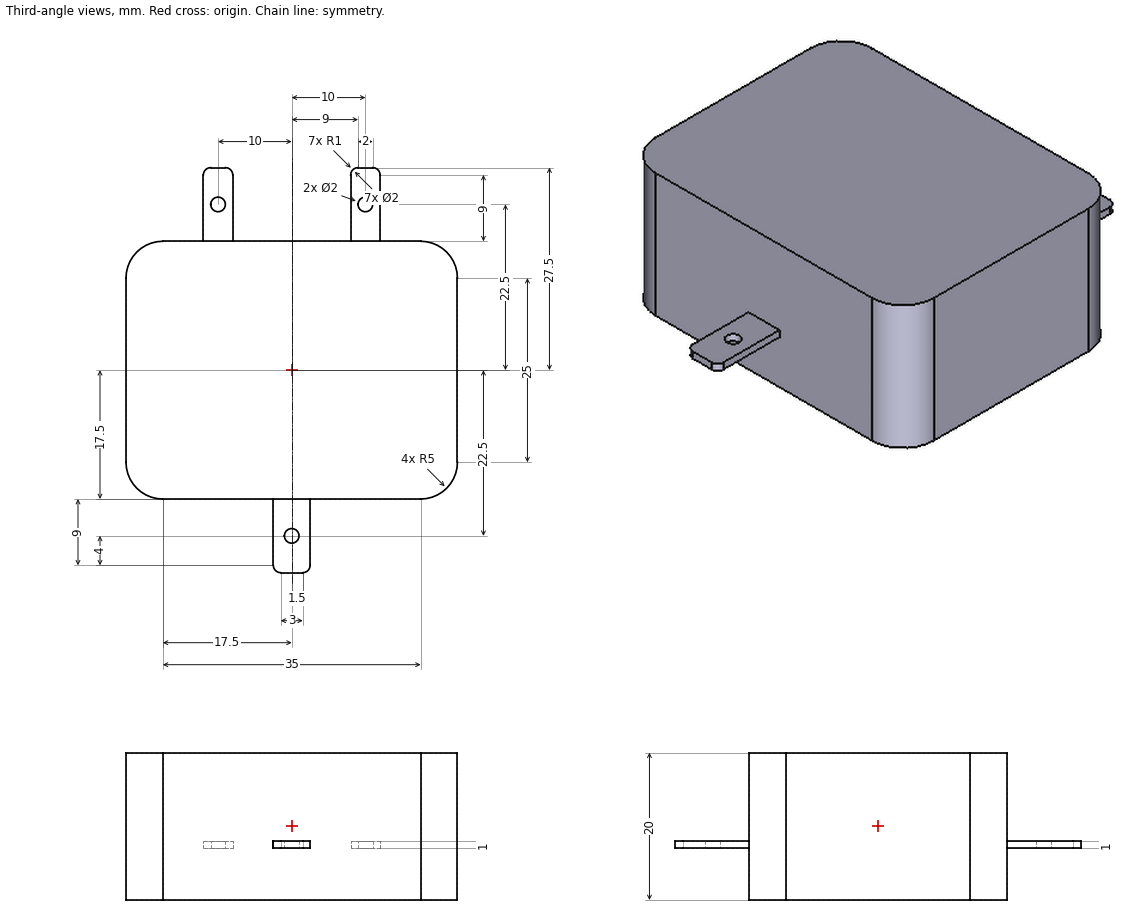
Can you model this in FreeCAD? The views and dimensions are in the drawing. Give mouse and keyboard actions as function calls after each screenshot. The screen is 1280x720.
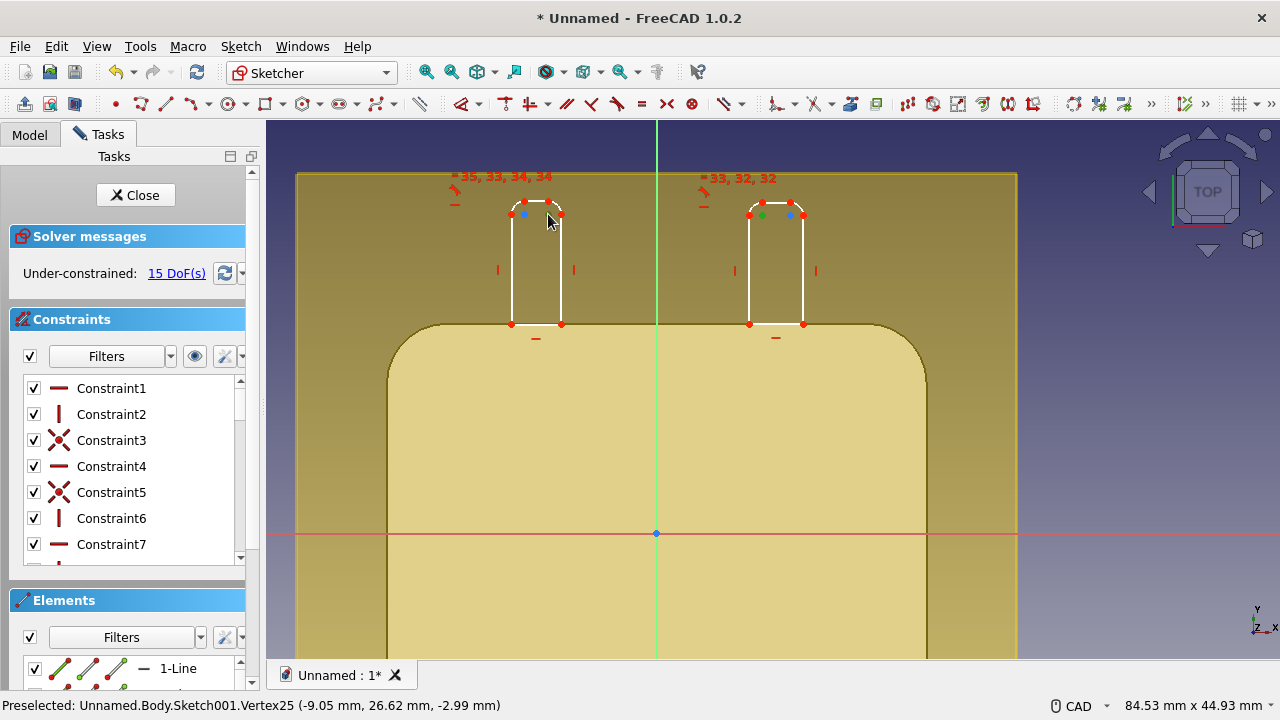
click(657, 596)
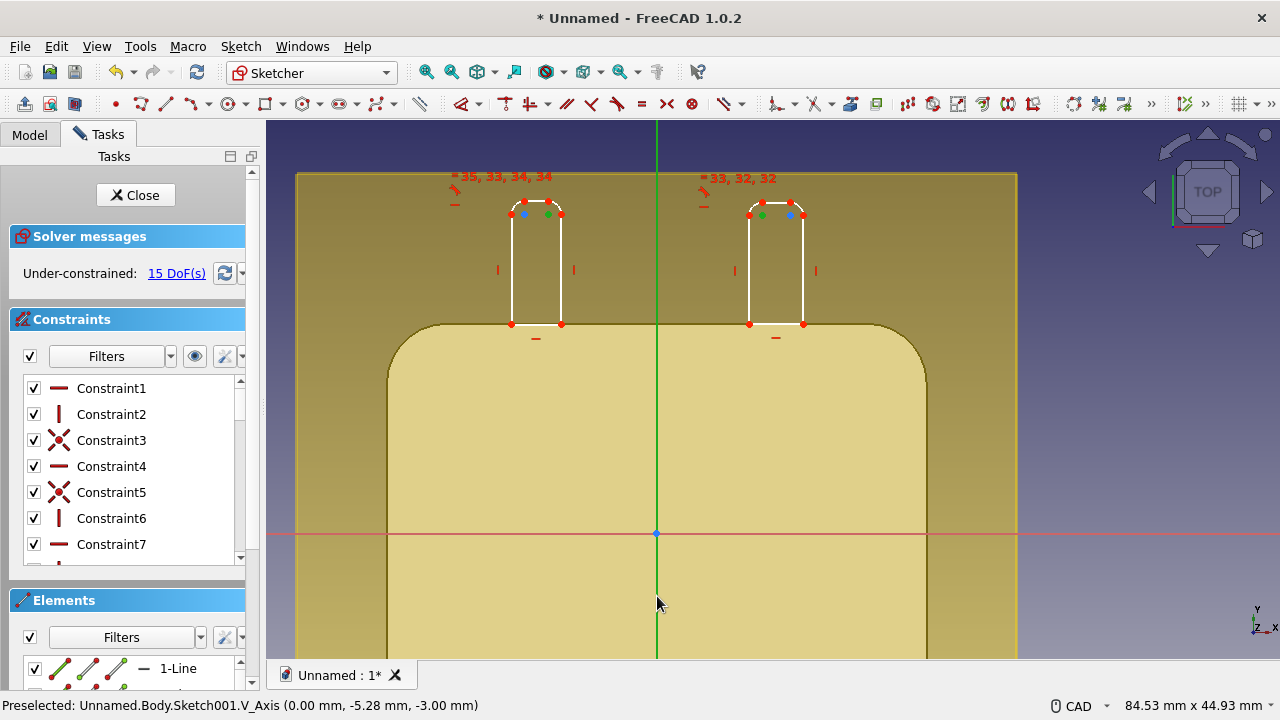
click(667, 104)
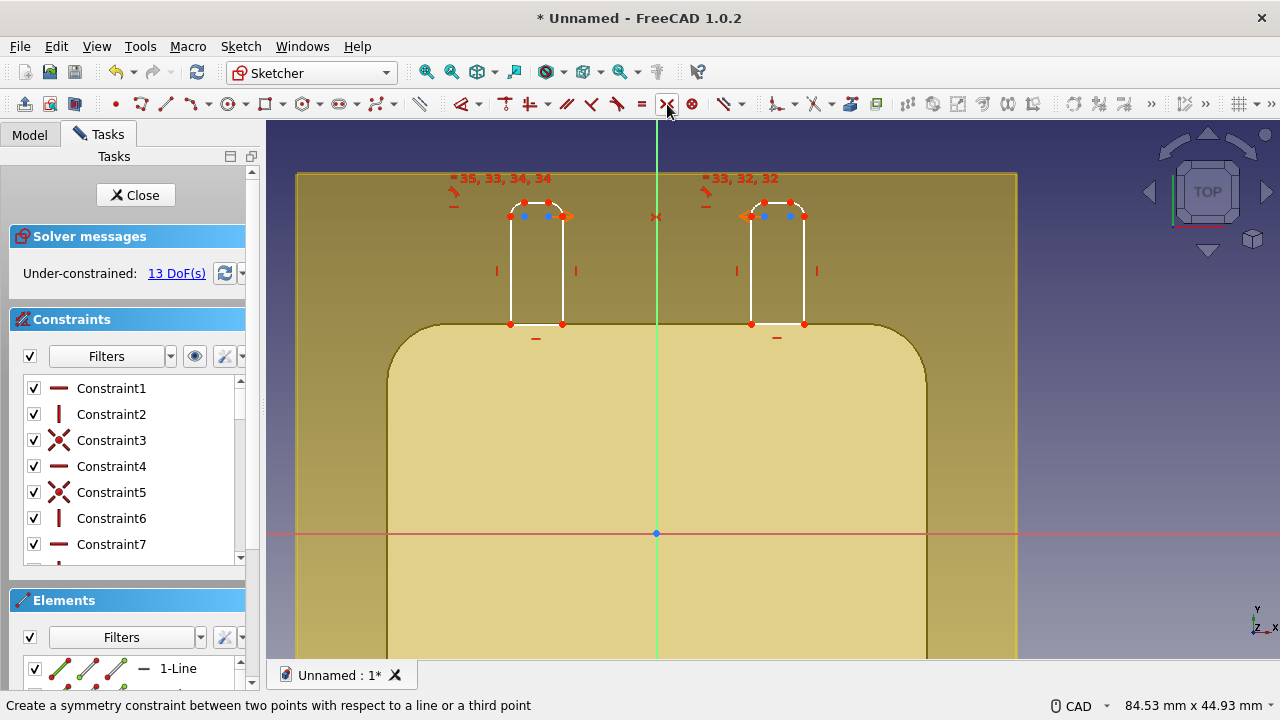
click(804, 324)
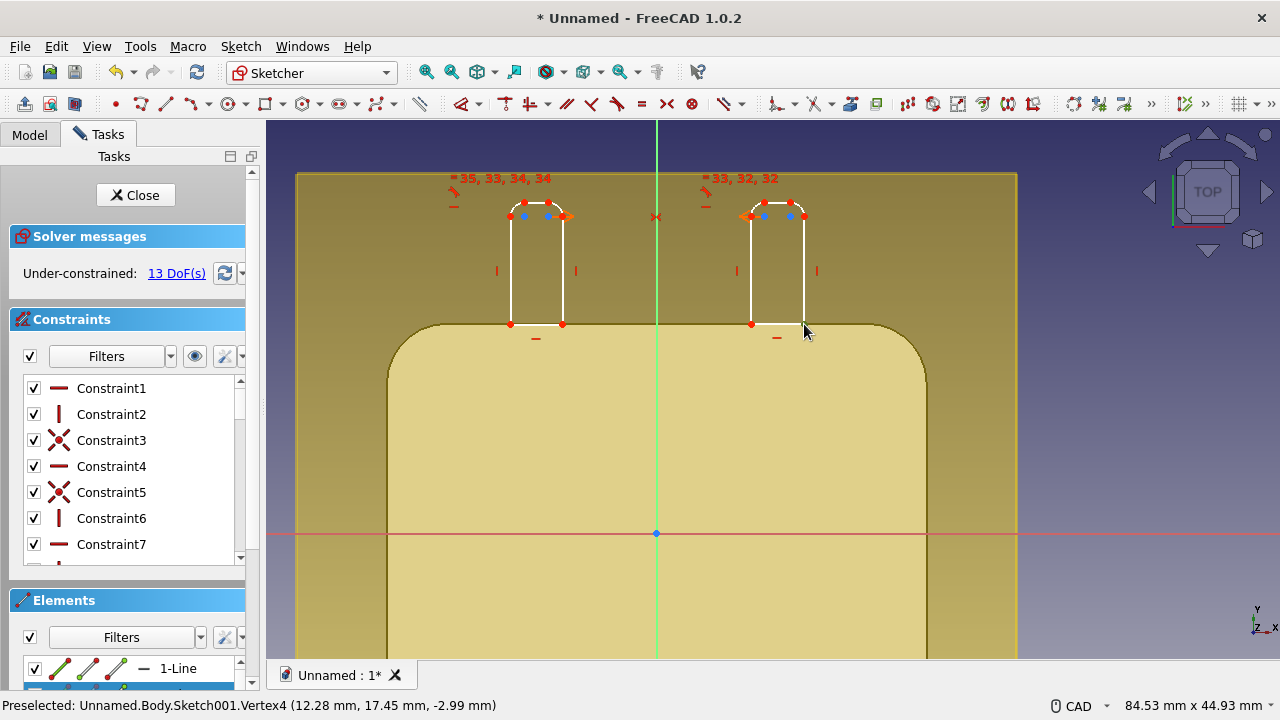
click(511, 325)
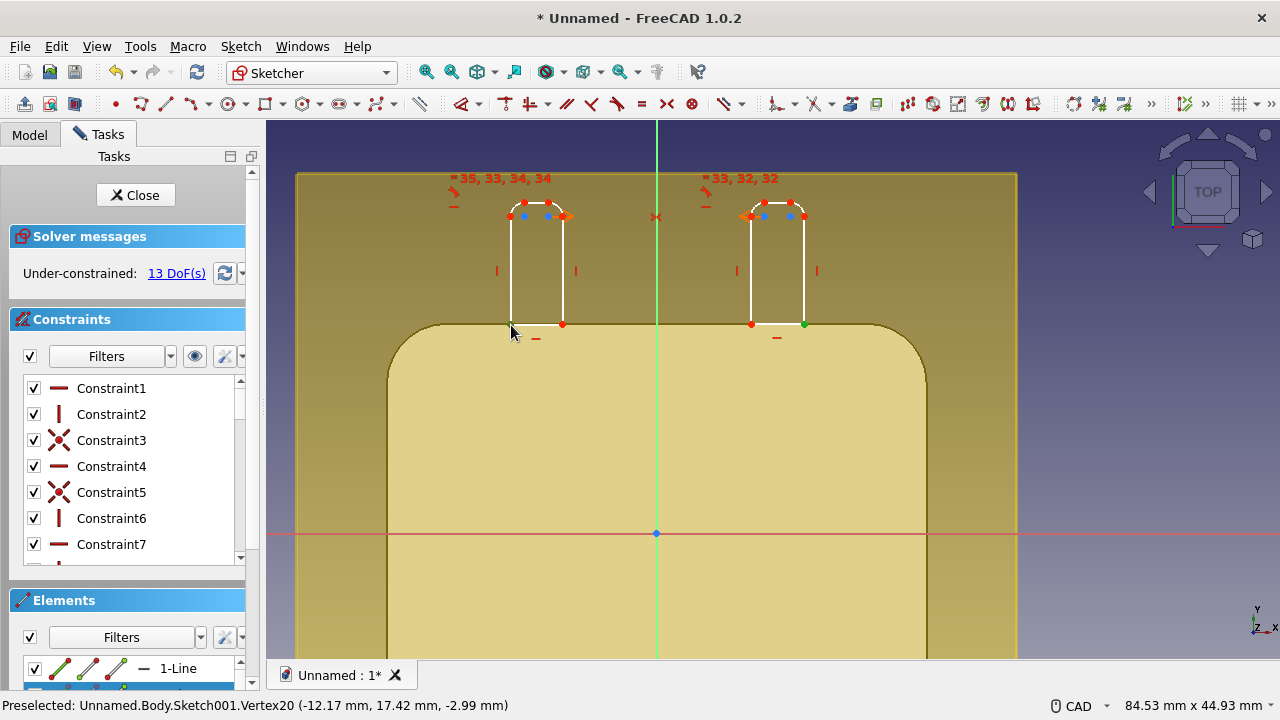
click(657, 596)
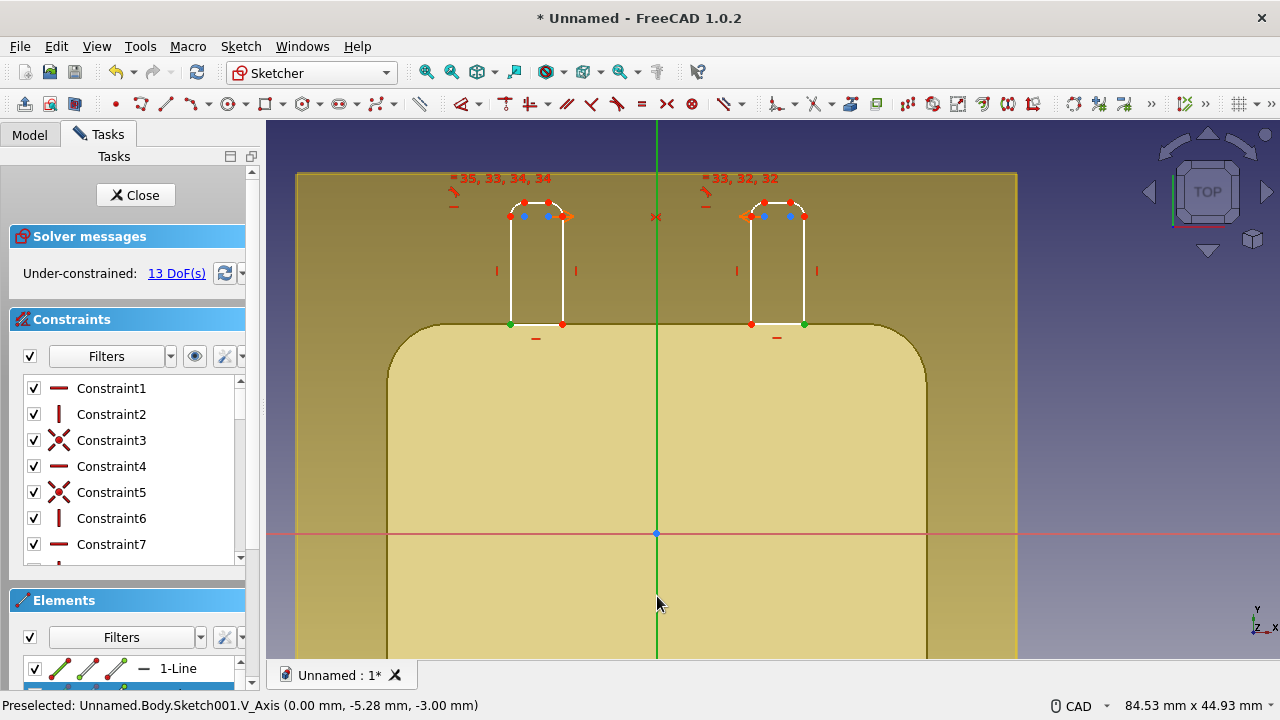
key(s)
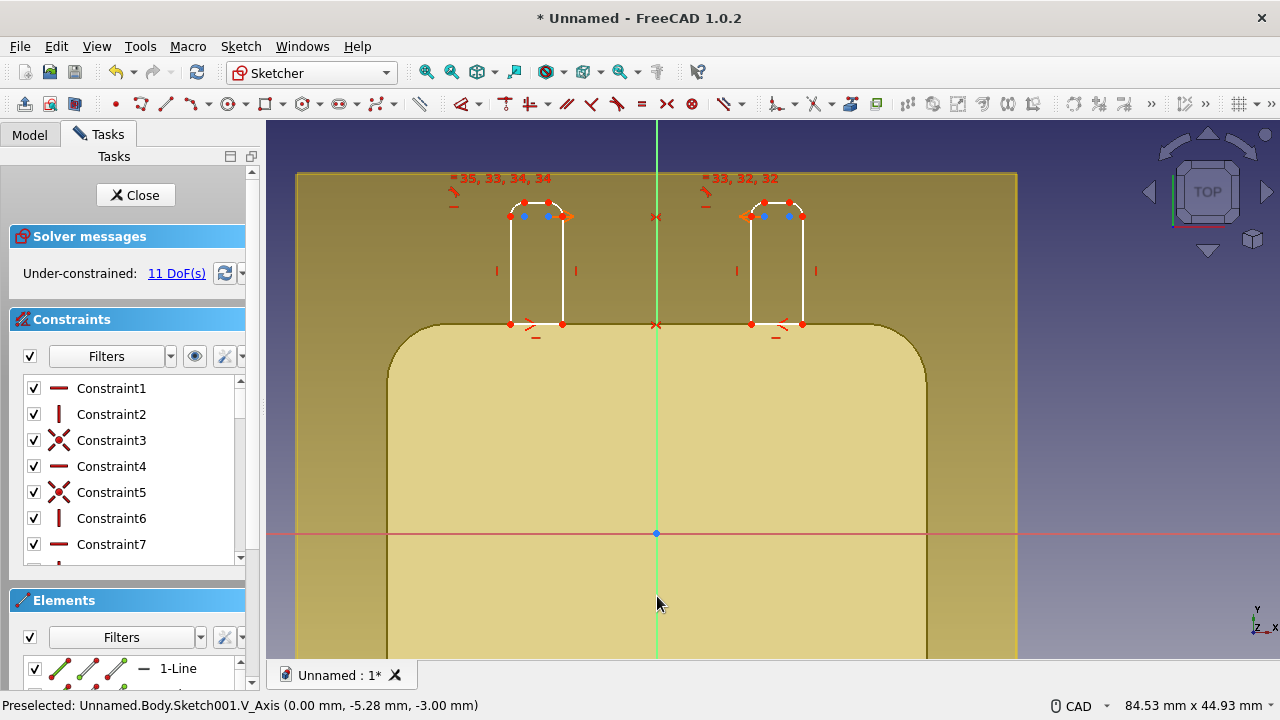
key(d)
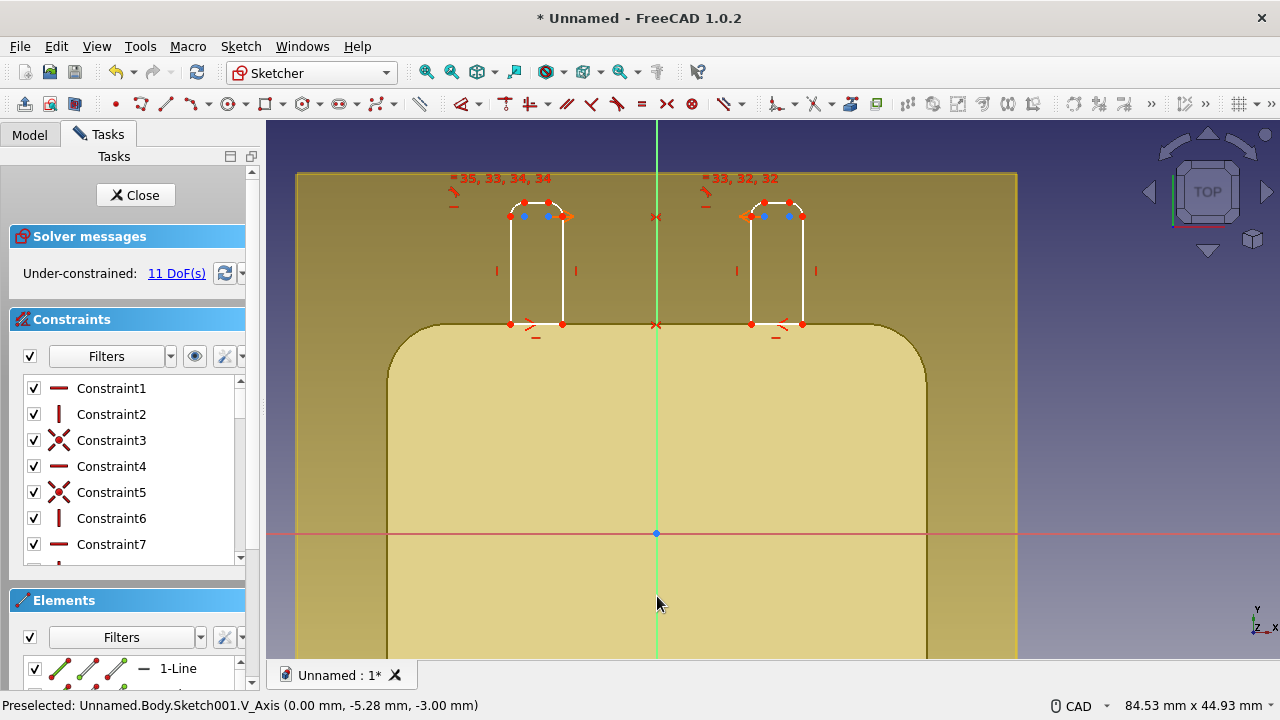
scroll(799, 207, up, 6)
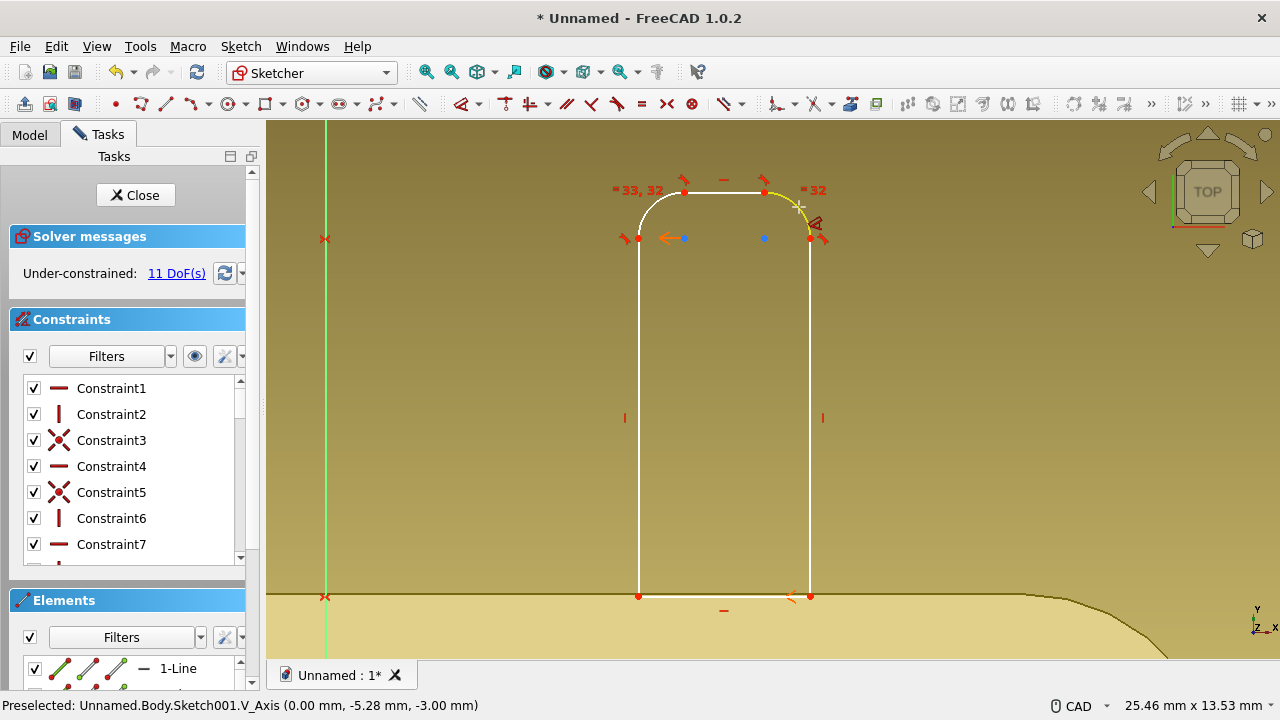
click(797, 206)
click(820, 183)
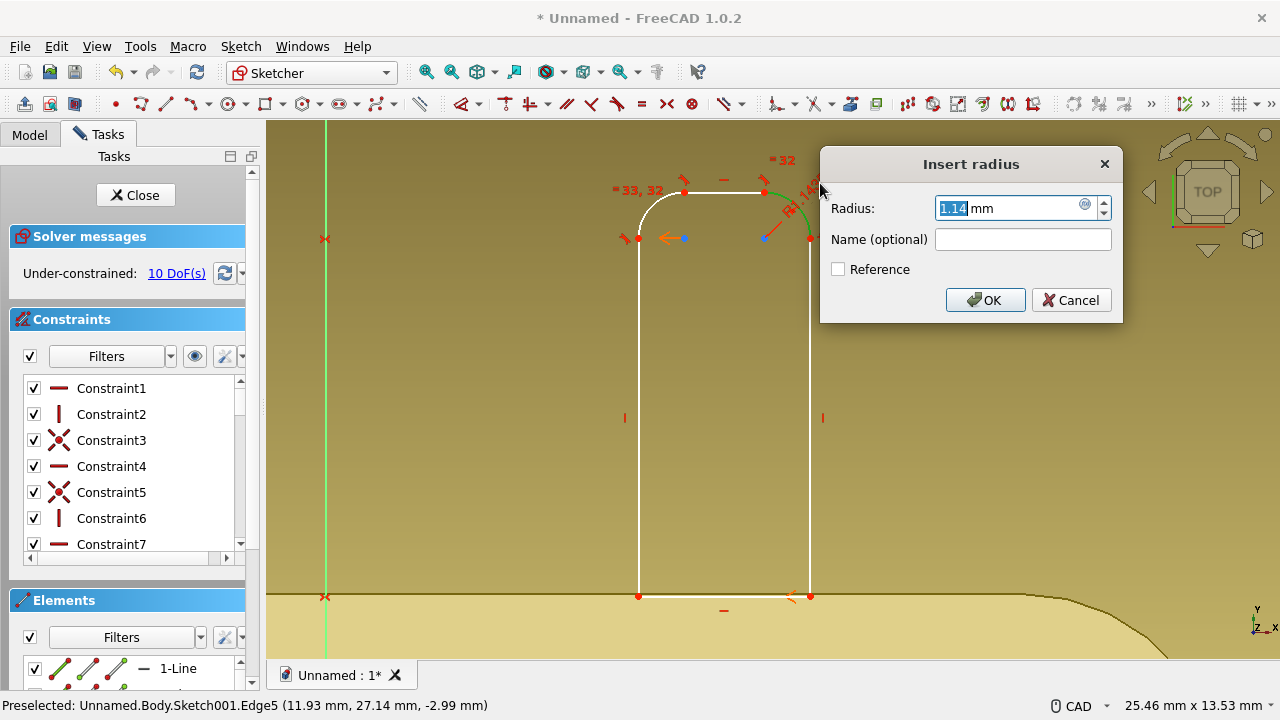
text(1)
key(Return)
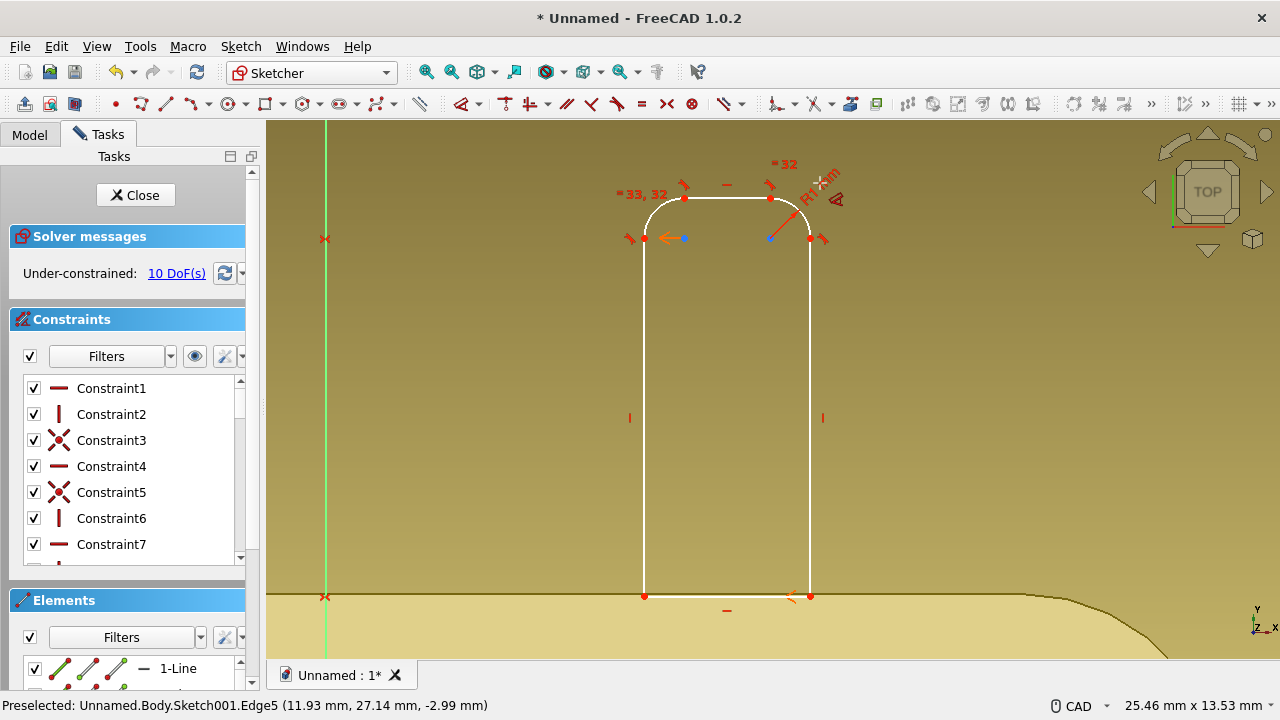
scroll(780, 211, down, 9)